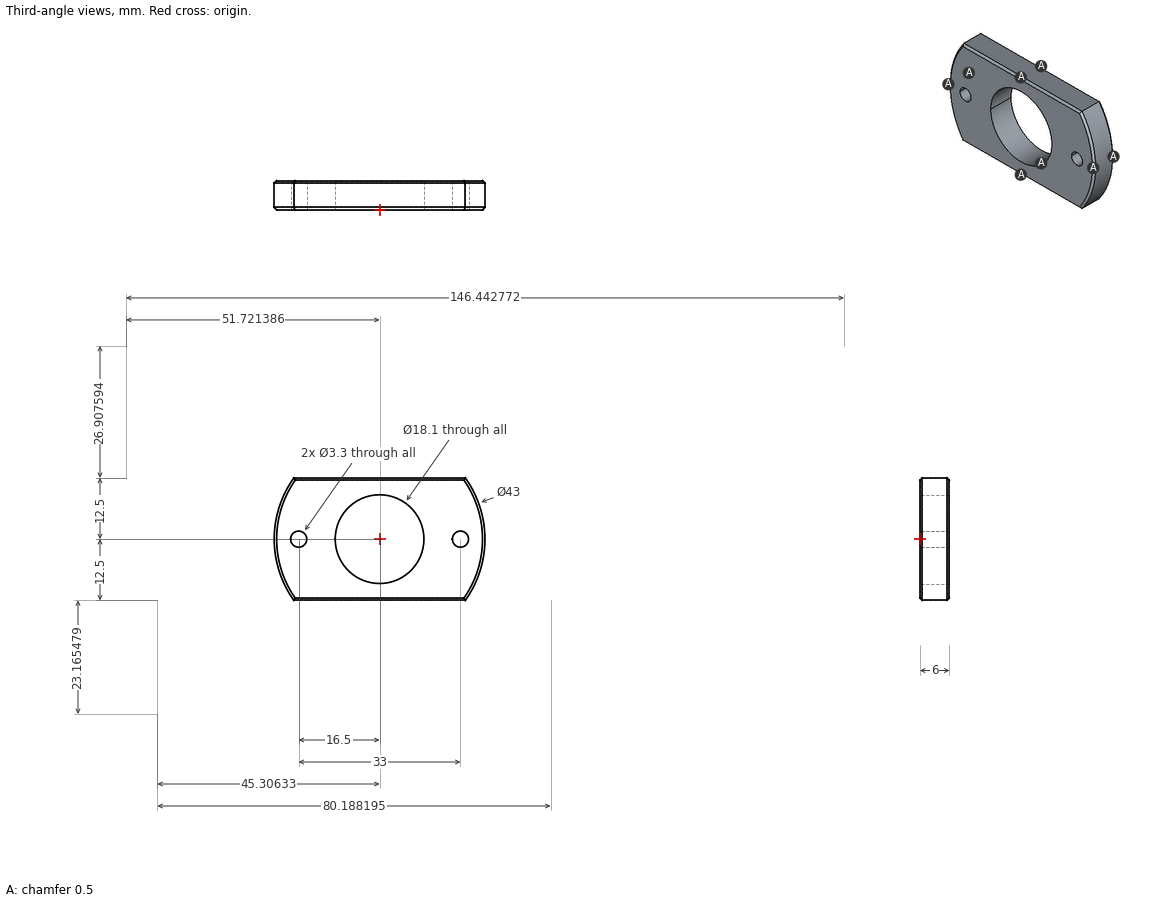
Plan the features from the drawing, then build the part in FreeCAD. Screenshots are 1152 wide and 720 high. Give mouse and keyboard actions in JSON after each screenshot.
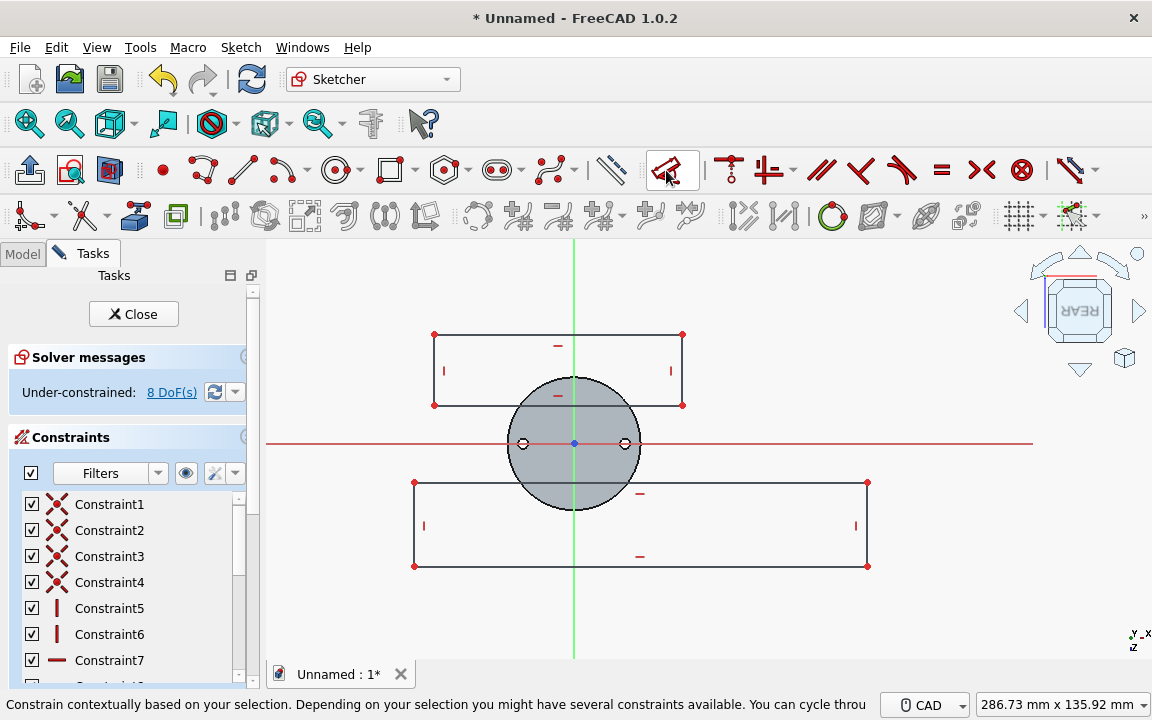
{"action": "left_click", "coordinate": [434, 406]}
{"action": "left_click", "coordinate": [400, 425]}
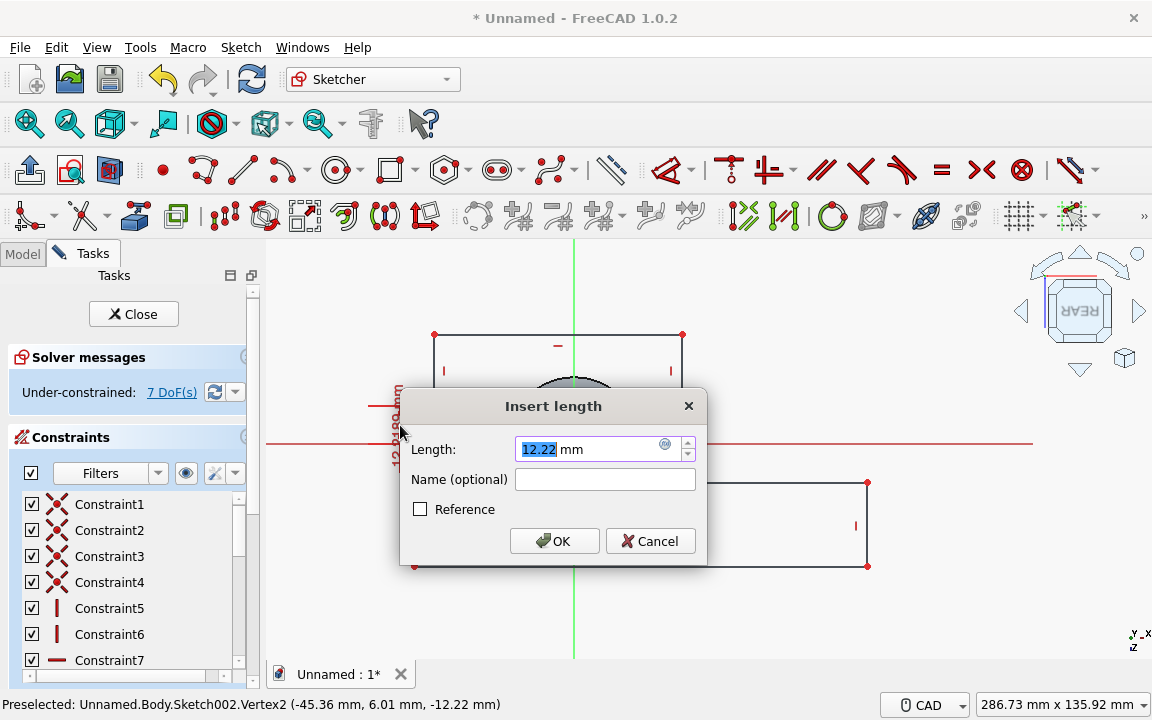
{"action": "type", "text": "12.5"}
{"action": "key", "text": "Return"}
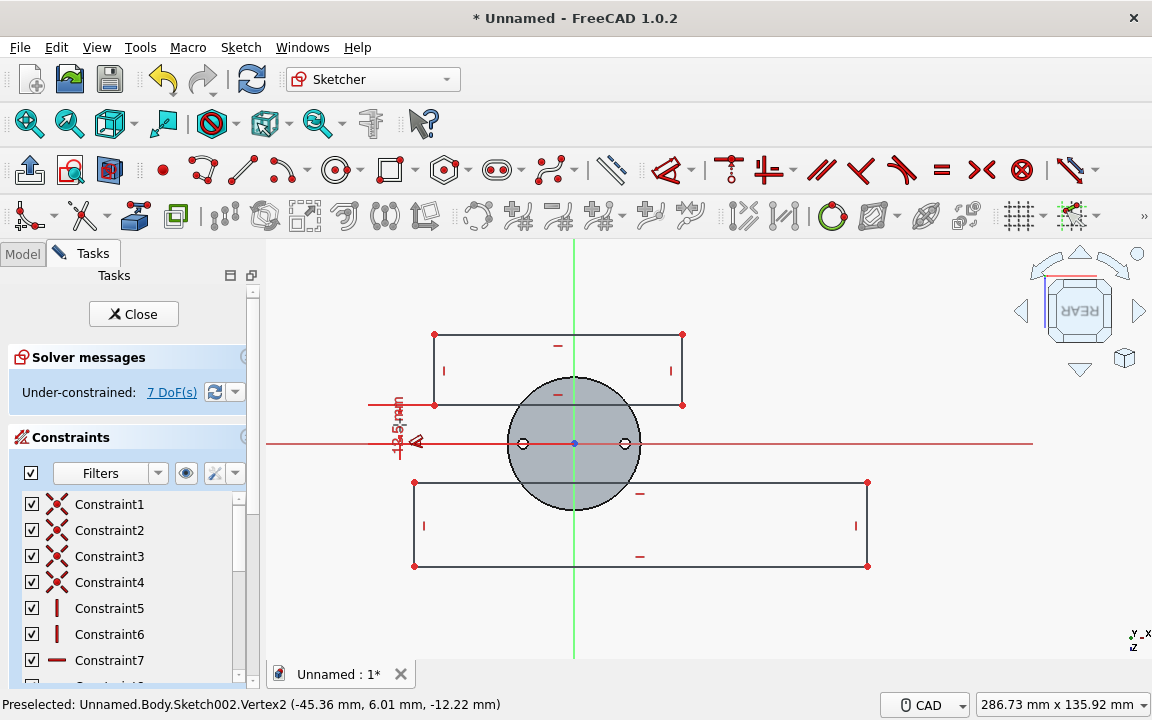
{"action": "left_click", "coordinate": [414, 483]}
{"action": "left_click", "coordinate": [380, 463]}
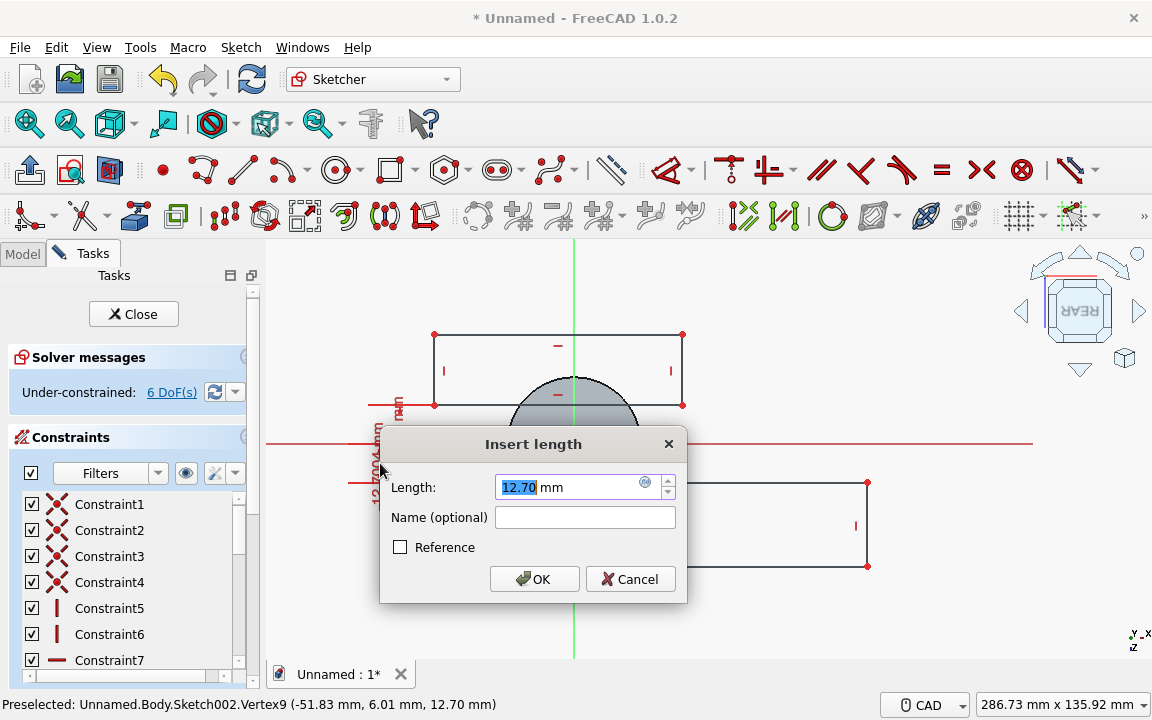
{"action": "type", "text": "12.5"}
{"action": "key", "text": "Return"}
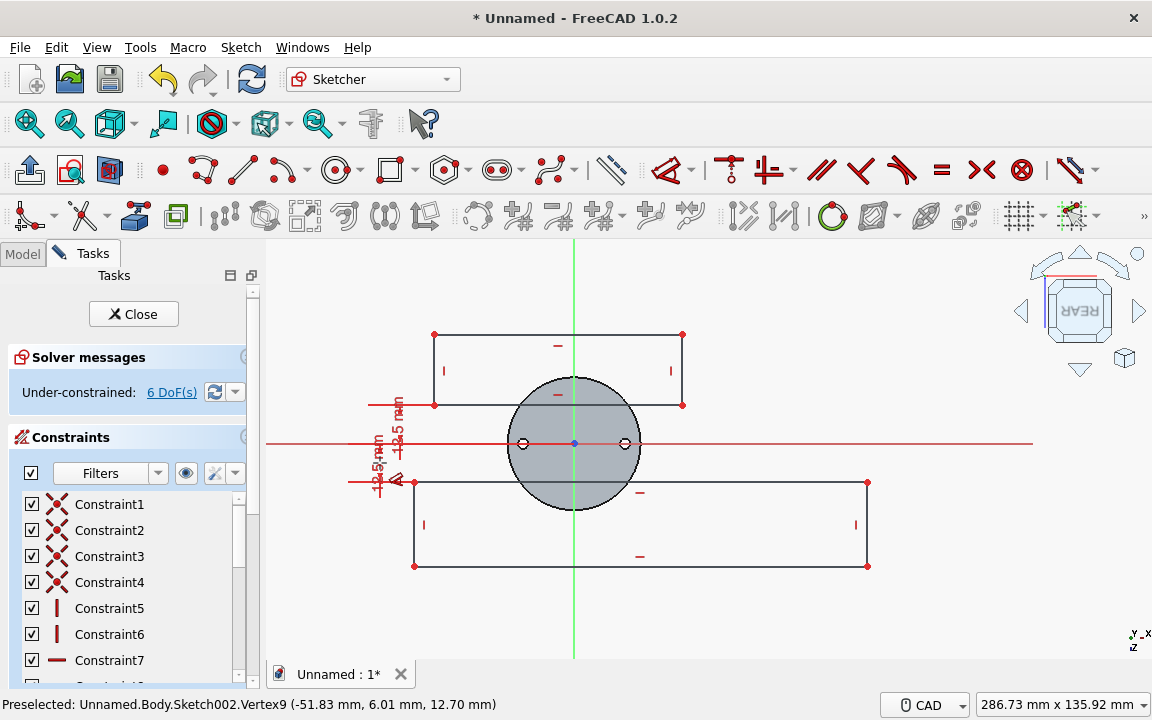
{"action": "left_click", "coordinate": [434, 356]}
{"action": "left_click", "coordinate": [400, 370]}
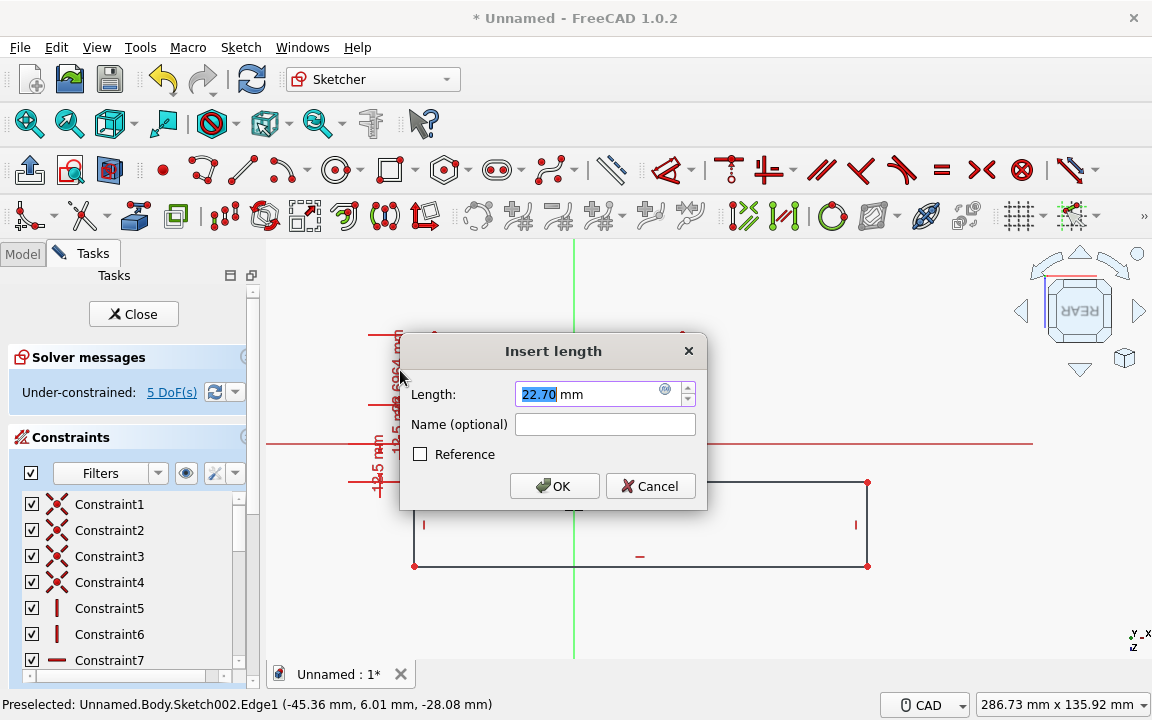
{"action": "type", "text": "23.165479"}
{"action": "key", "text": "Return"}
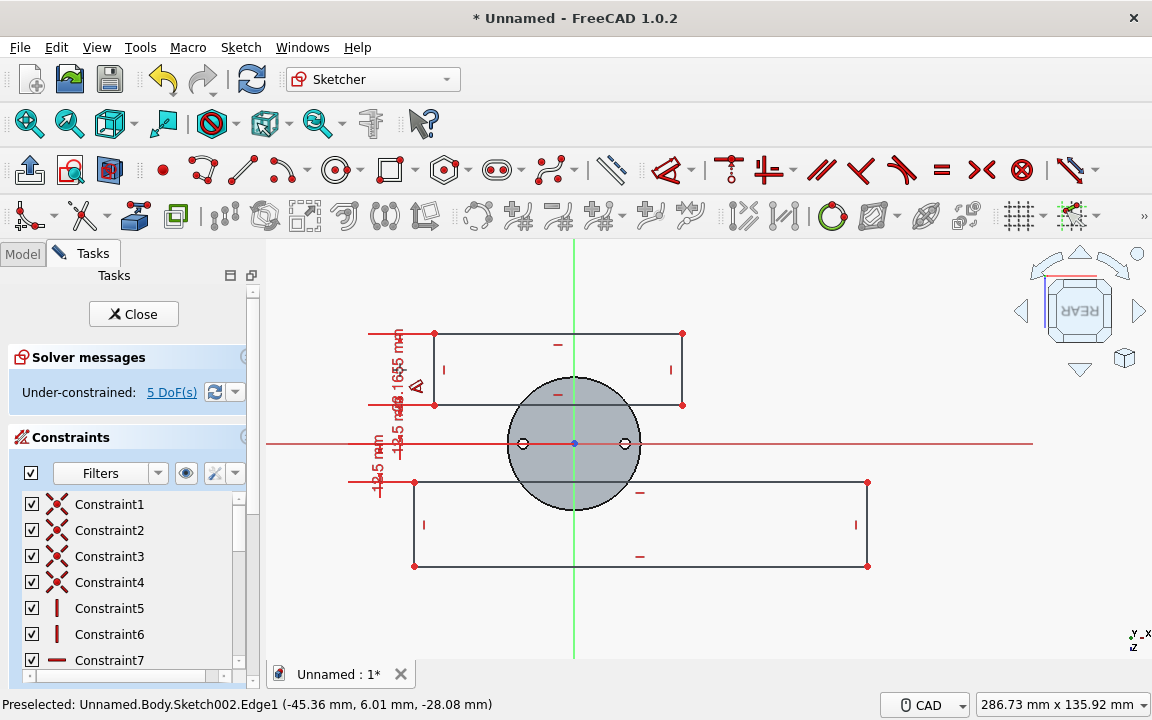
{"action": "left_click", "coordinate": [508, 405]}
{"action": "left_click", "coordinate": [558, 371]}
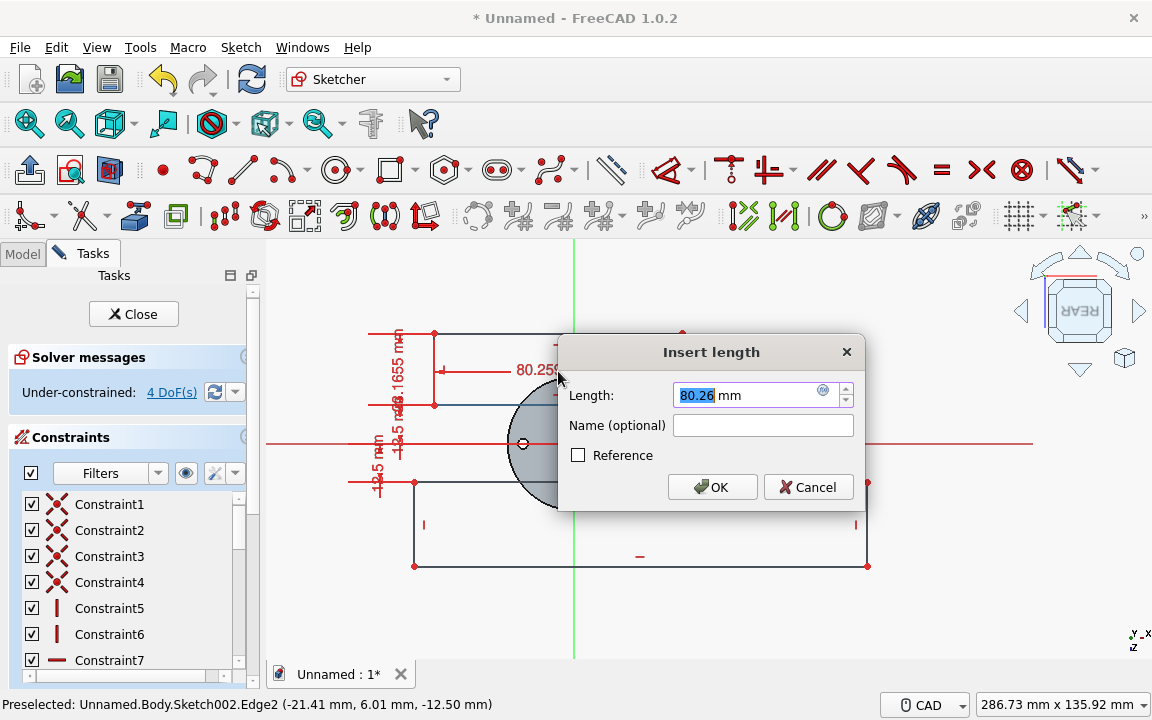
{"action": "type", "text": "80.188195"}
{"action": "key", "text": "Return"}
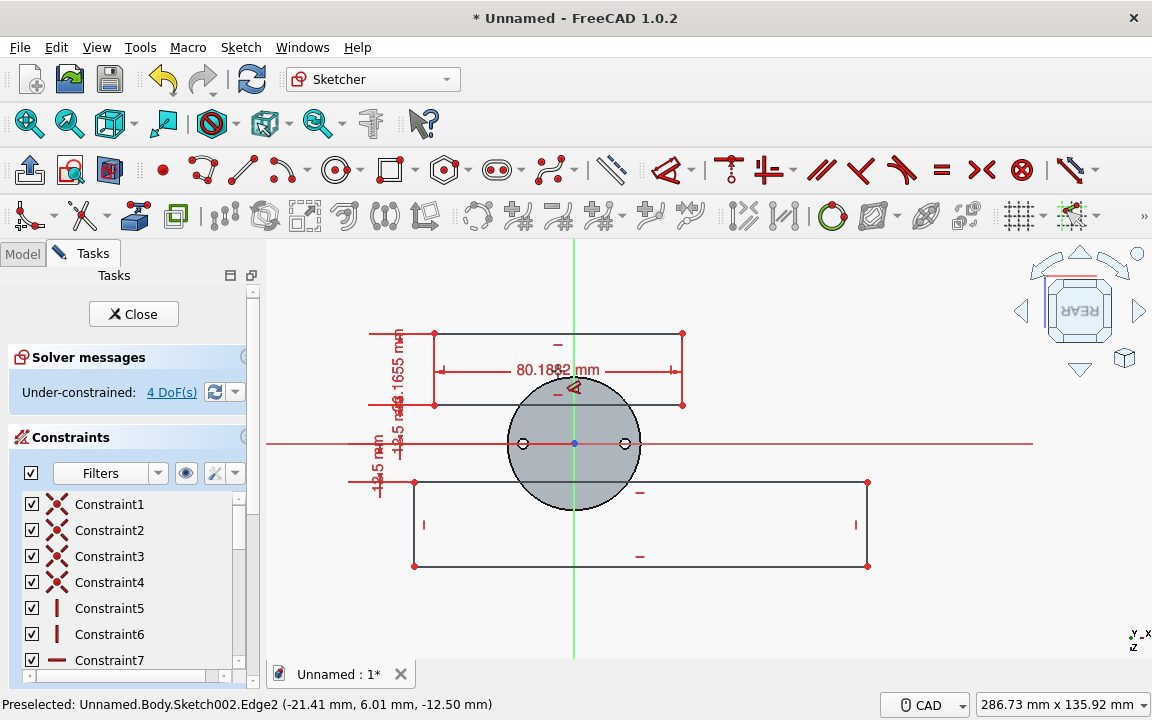
{"action": "left_click", "coordinate": [414, 508]}
{"action": "left_click", "coordinate": [380, 525]}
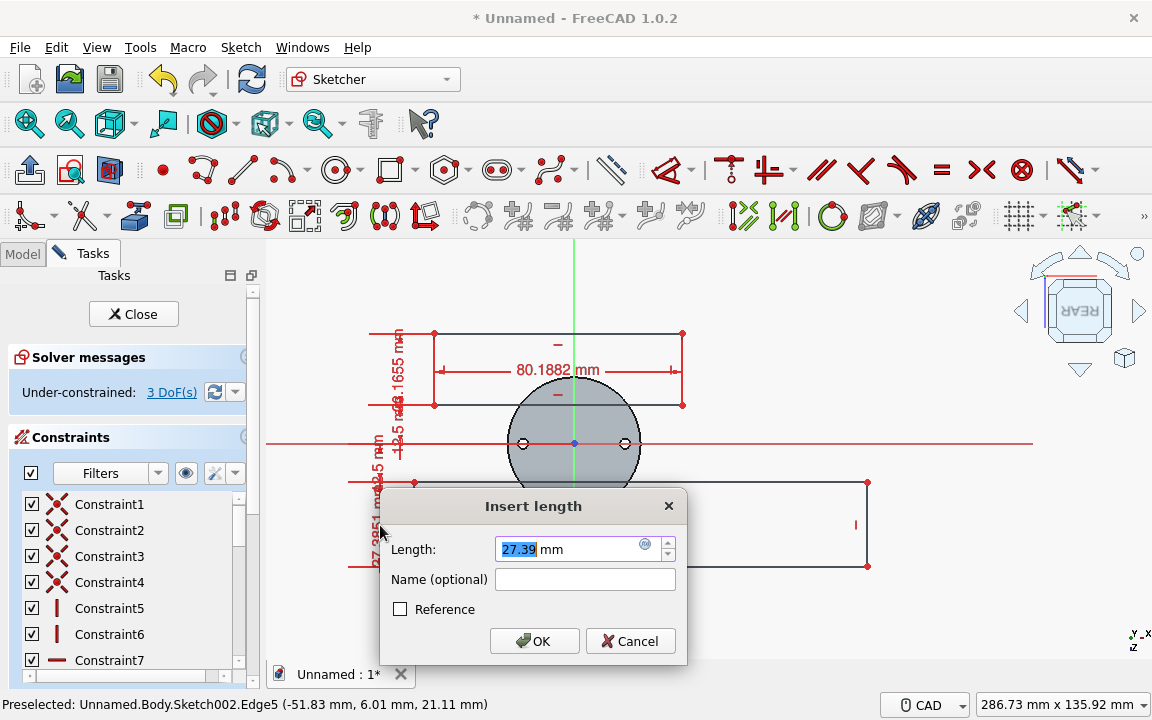
{"action": "type", "text": "26.907594"}
{"action": "key", "text": "Return"}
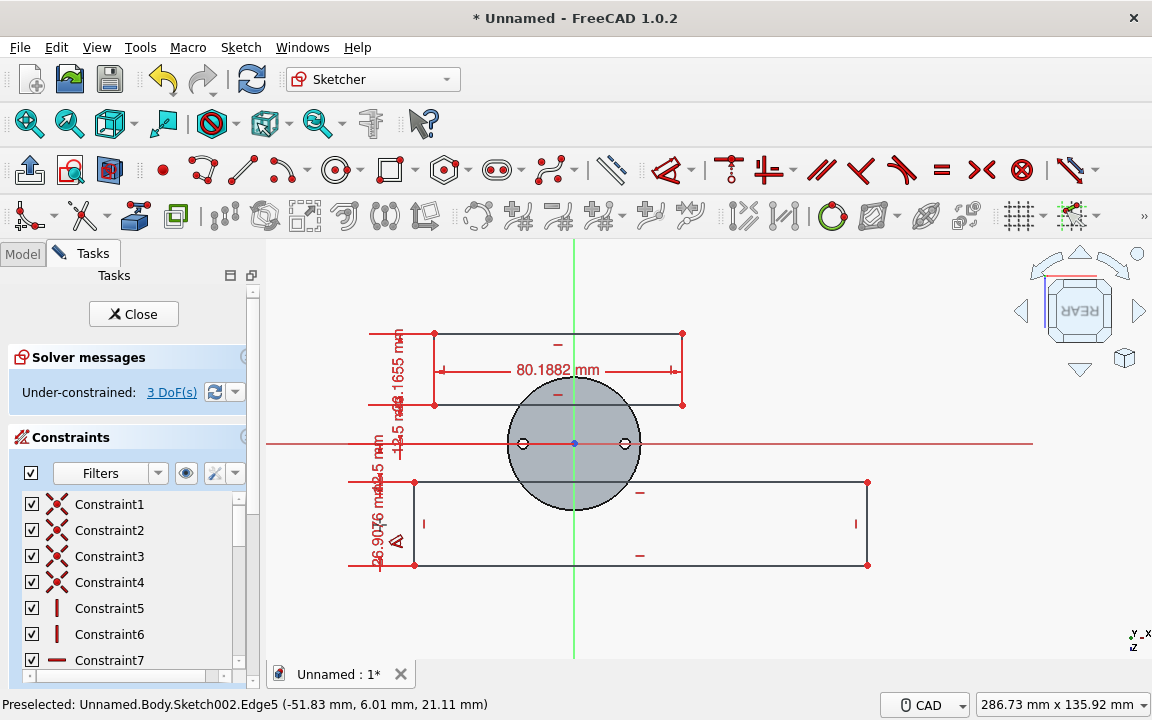
{"action": "left_click", "coordinate": [434, 334]}
{"action": "left_click", "coordinate": [504, 300]}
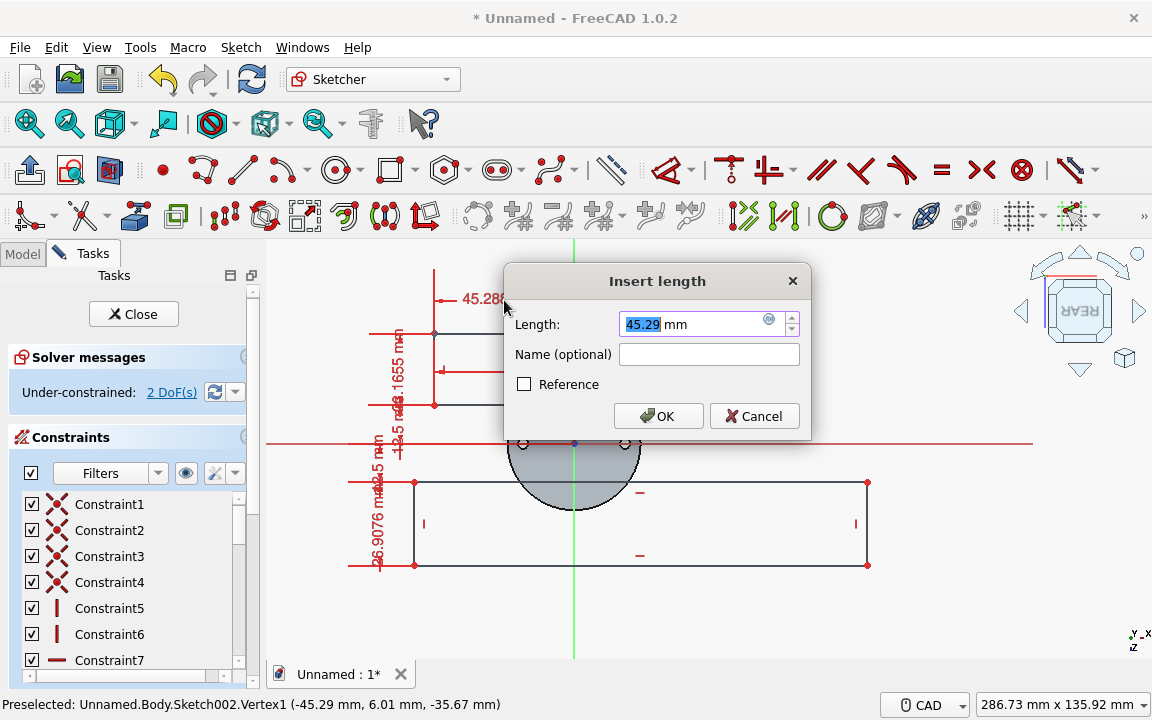
{"action": "type", "text": "45.30633"}
{"action": "key", "text": "Return"}